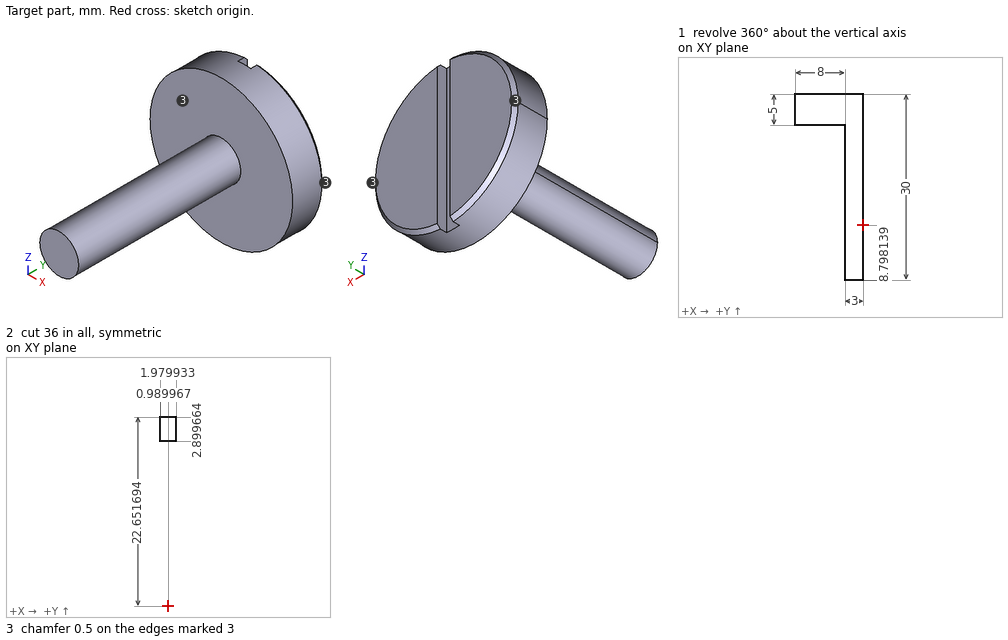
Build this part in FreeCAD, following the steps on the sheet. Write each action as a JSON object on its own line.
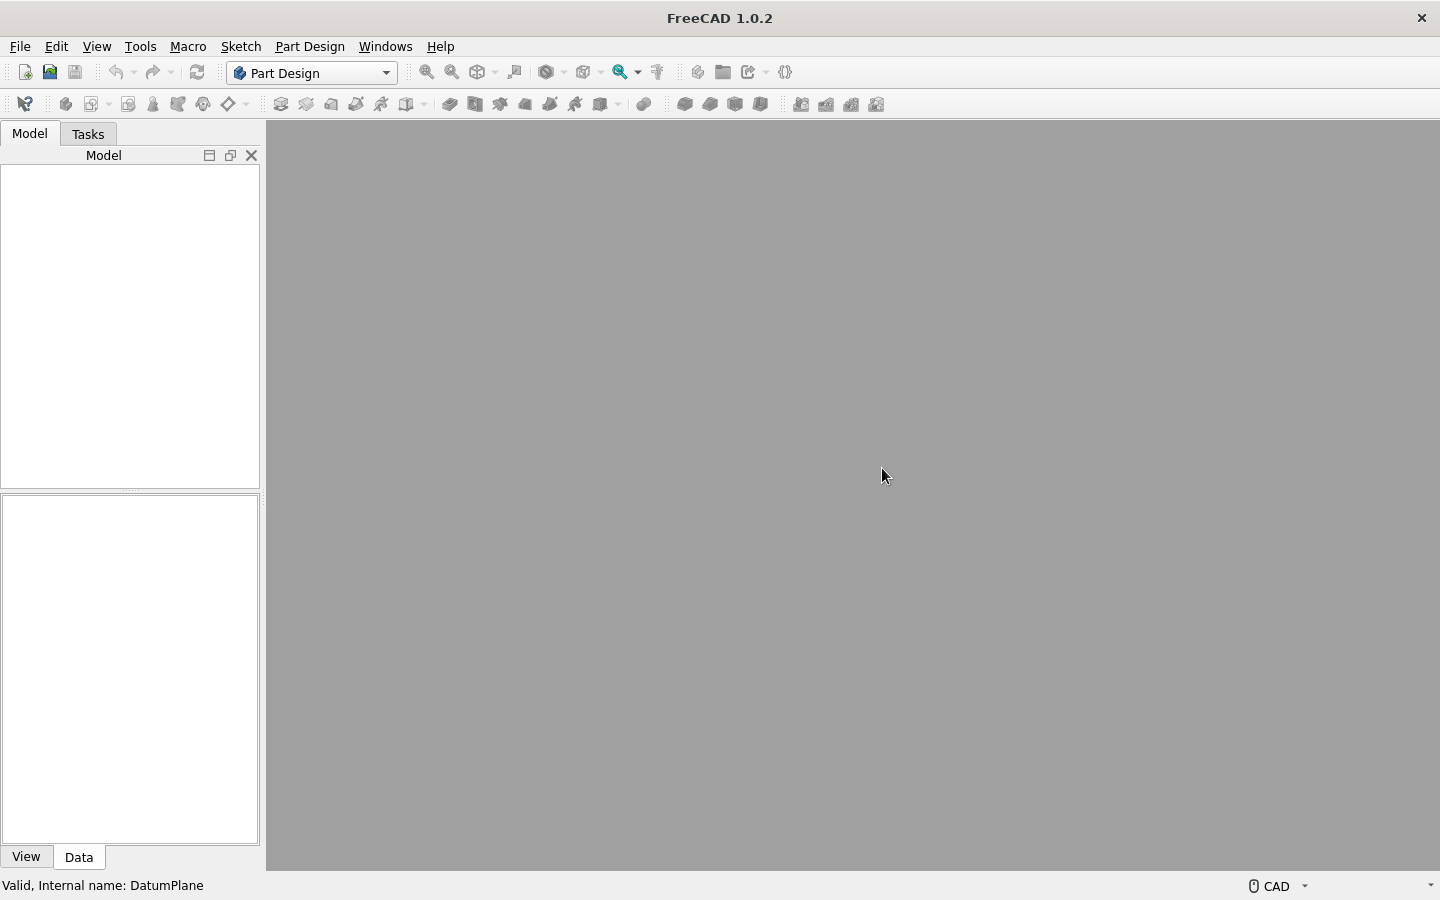
{"action": "left_click", "coordinate": [25, 72]}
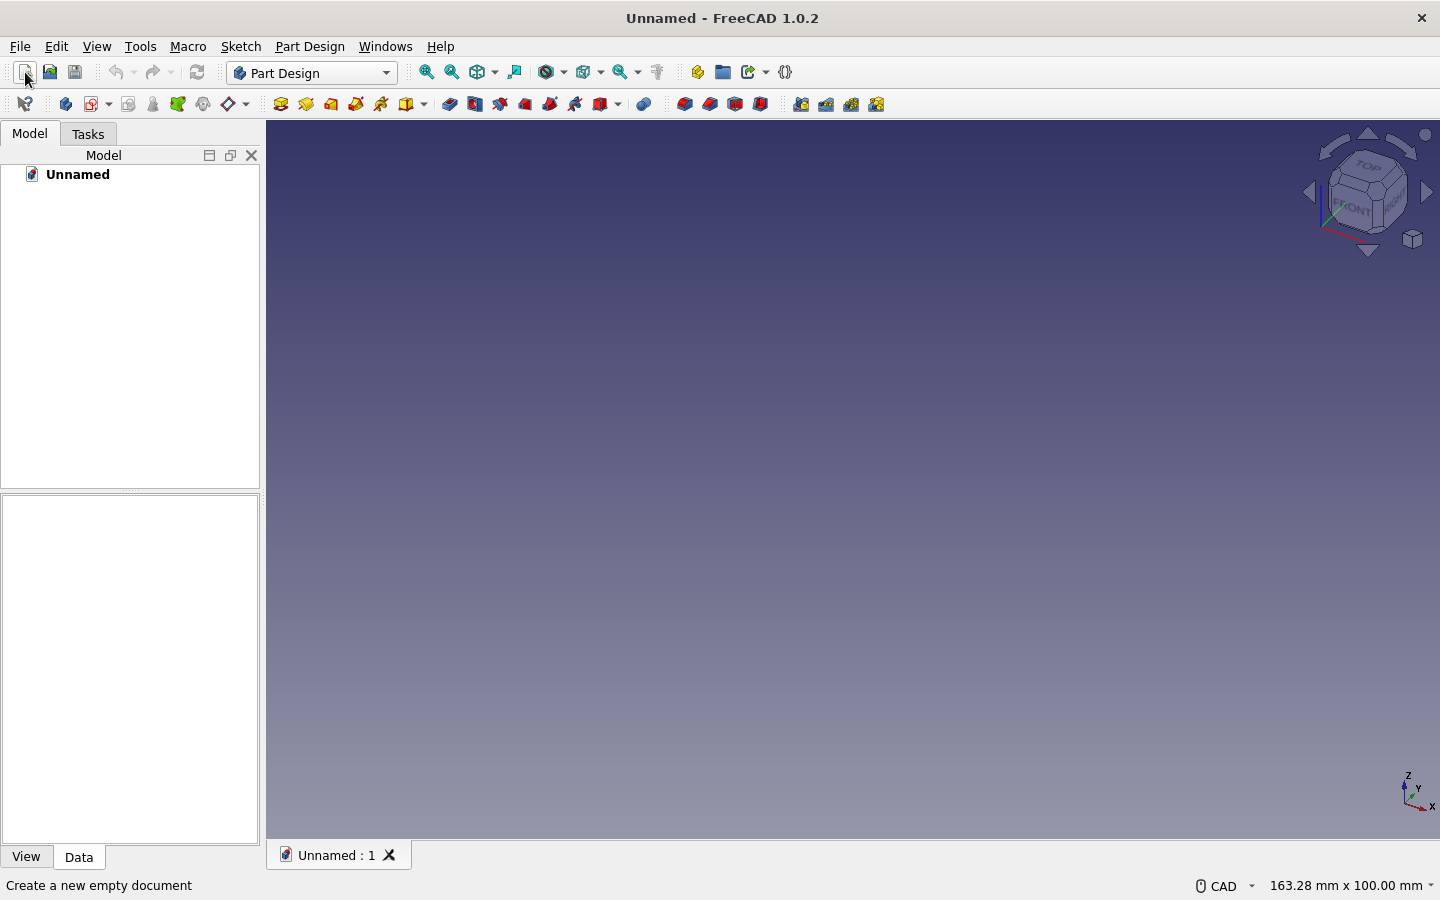
{"action": "left_click", "coordinate": [90, 104]}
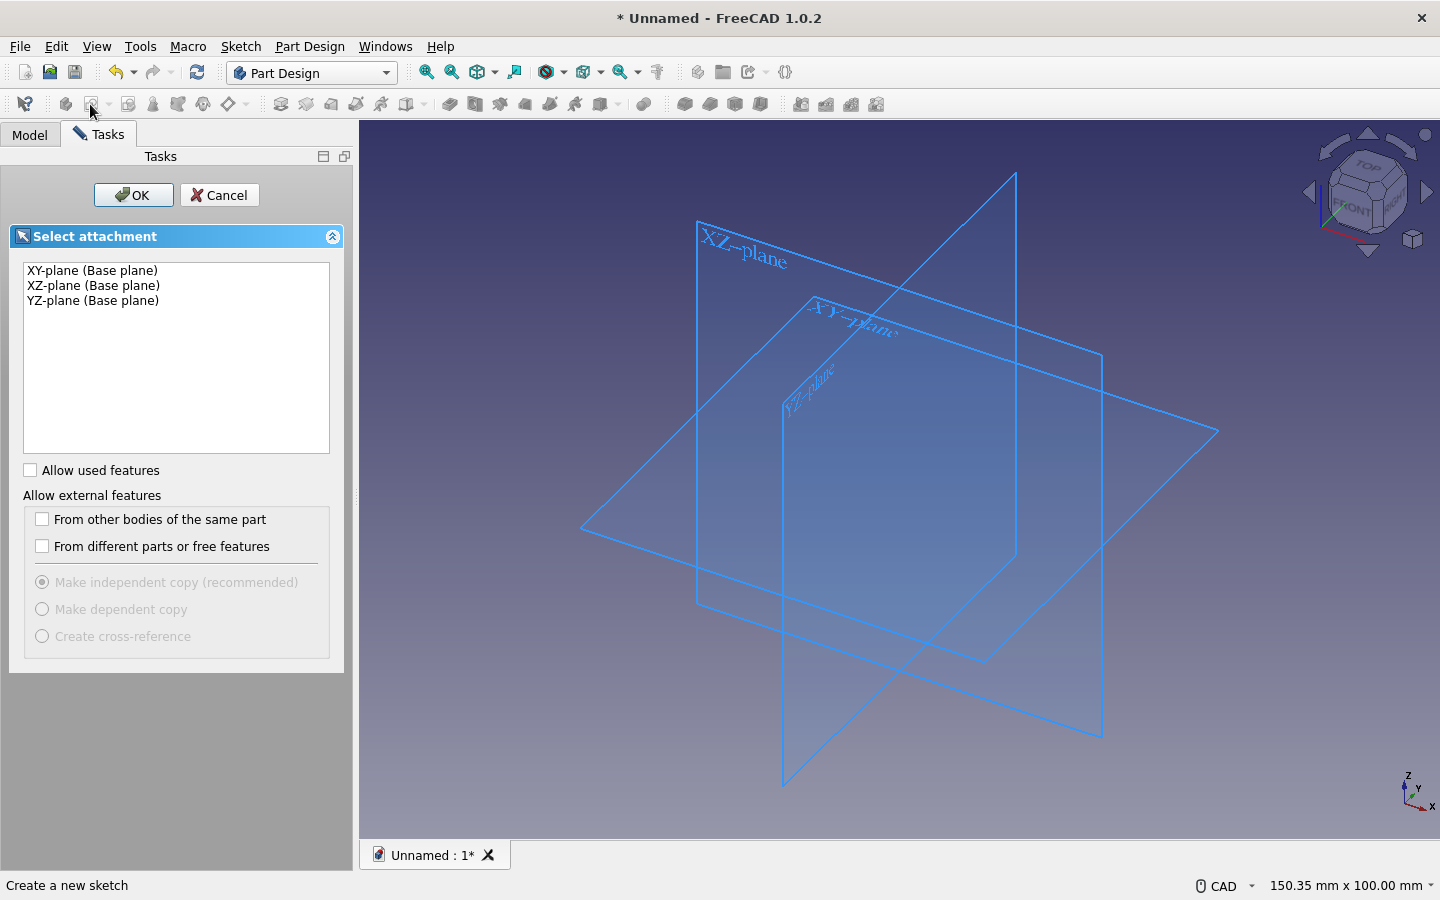
{"action": "left_click", "coordinate": [84, 270]}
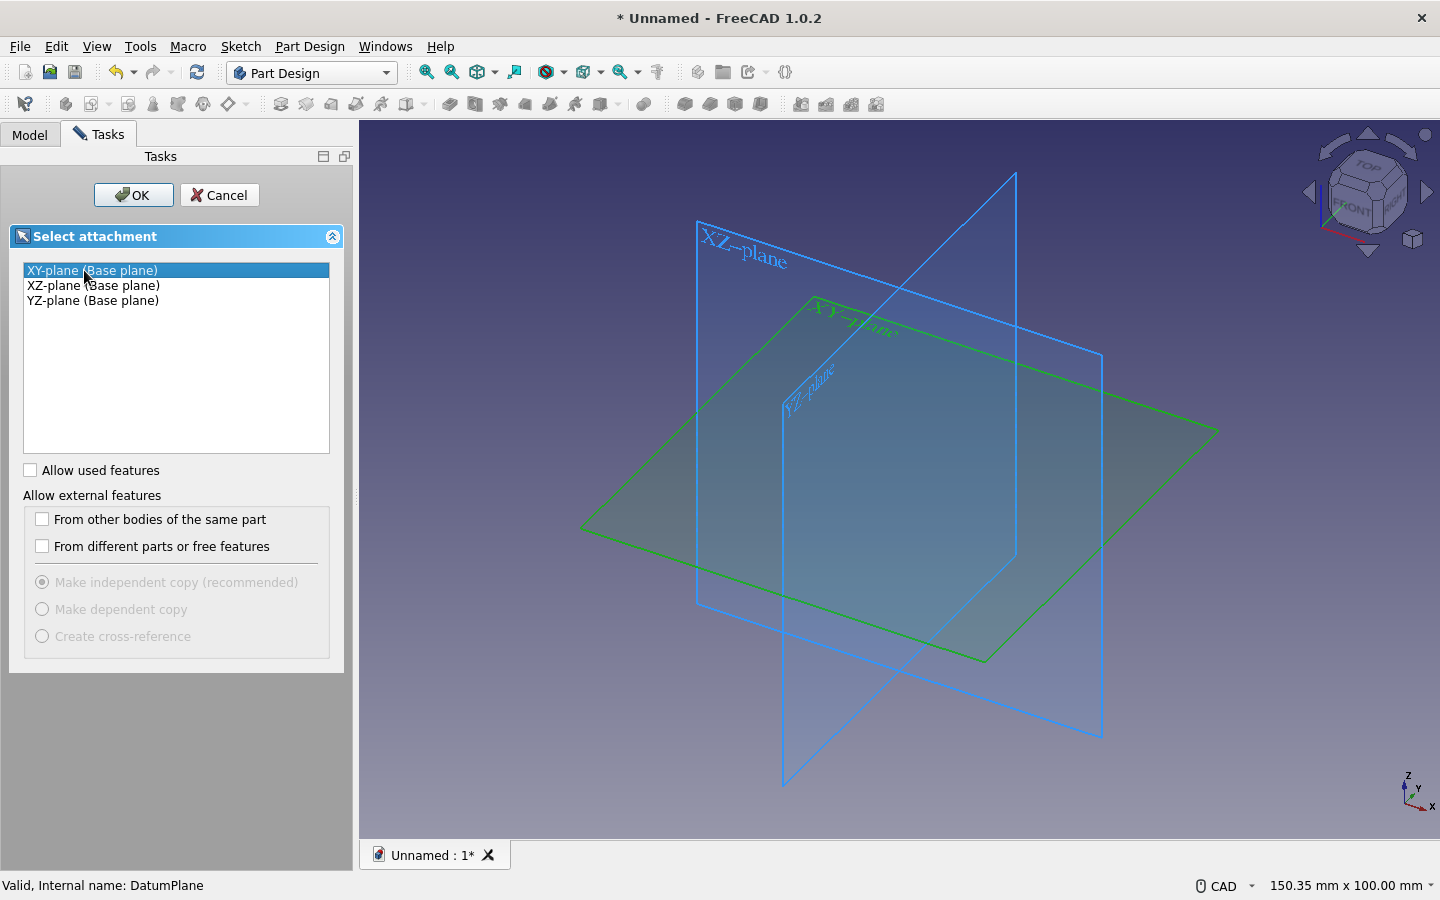
{"action": "left_click", "coordinate": [134, 195]}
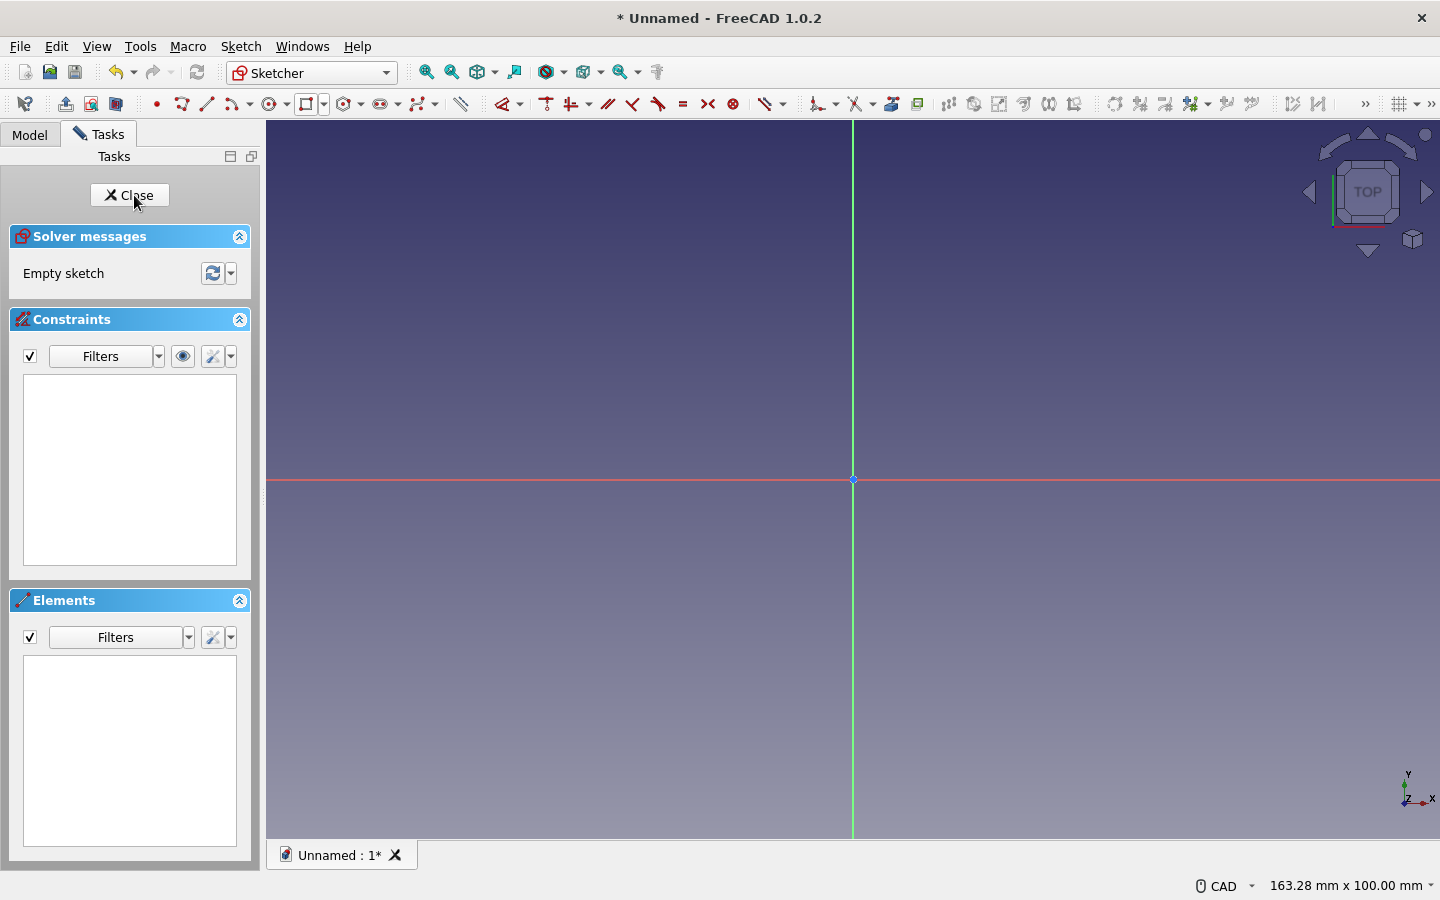
{"action": "scroll", "coordinate": [837, 399], "scroll_direction": "up", "scroll_amount": 4}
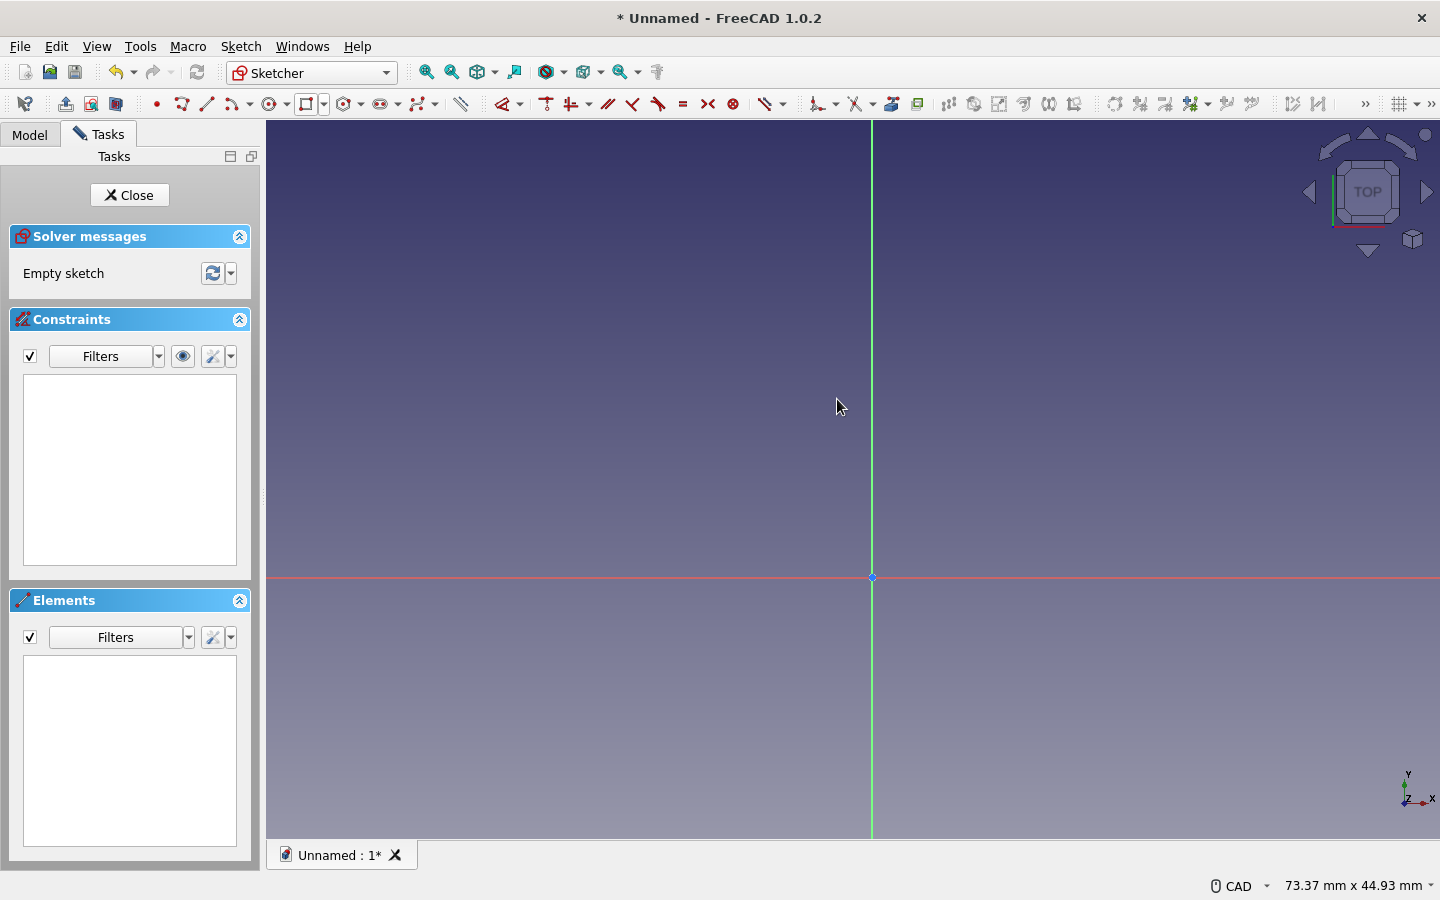
{"action": "left_click", "coordinate": [182, 104]}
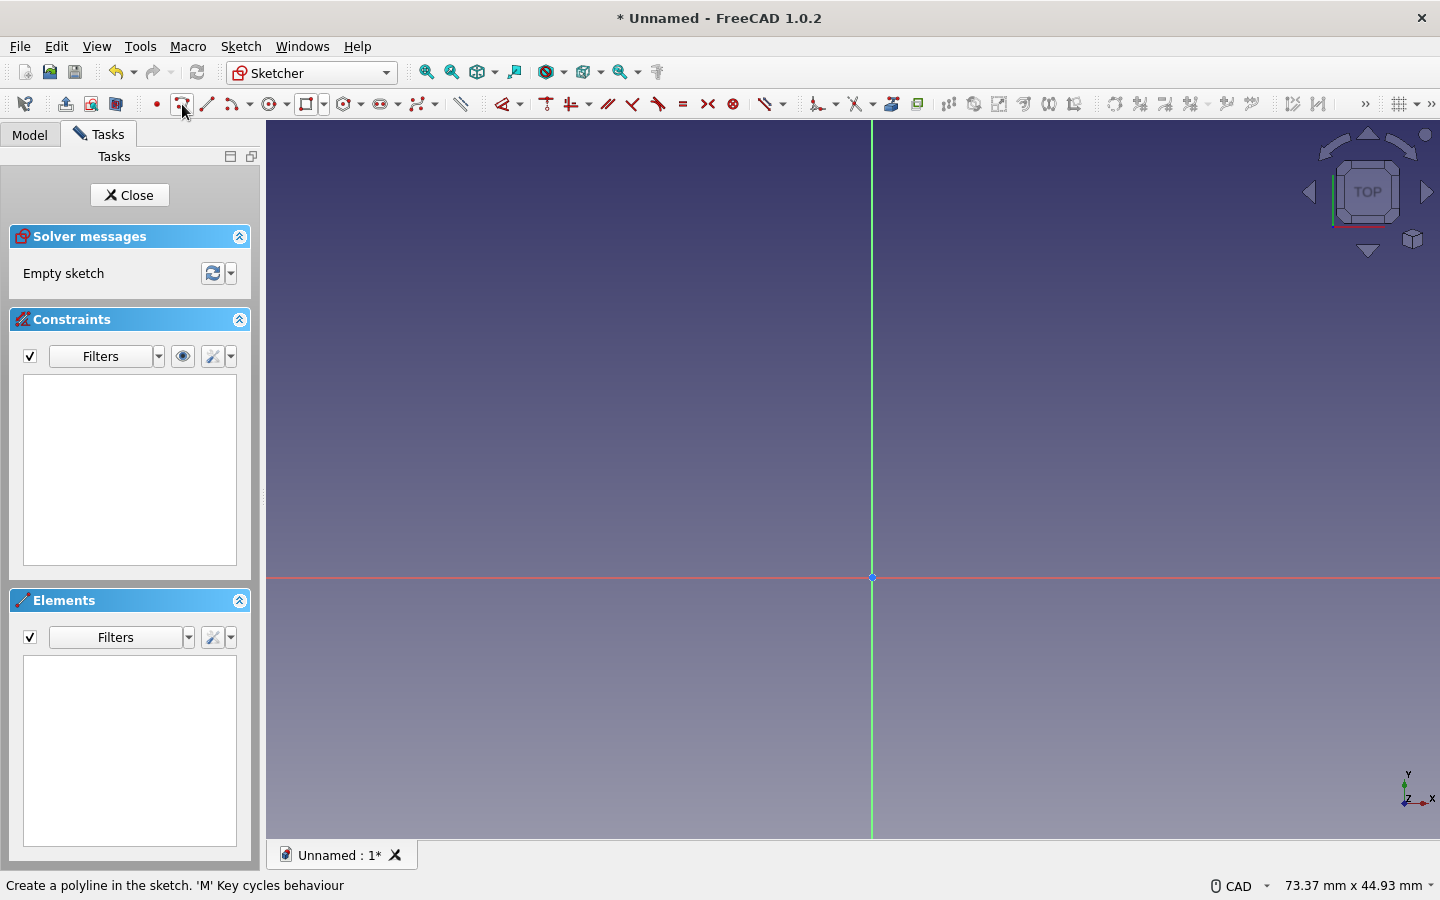
{"action": "left_click", "coordinate": [872, 718]}
{"action": "left_click", "coordinate": [863, 238]}
{"action": "left_click", "coordinate": [696, 238]}
{"action": "left_click", "coordinate": [696, 318]}
{"action": "left_click", "coordinate": [824, 318]}
{"action": "left_click", "coordinate": [824, 718]}
{"action": "left_click", "coordinate": [872, 719]}
{"action": "key", "text": "Escape"}
{"action": "key", "text": "Escape"}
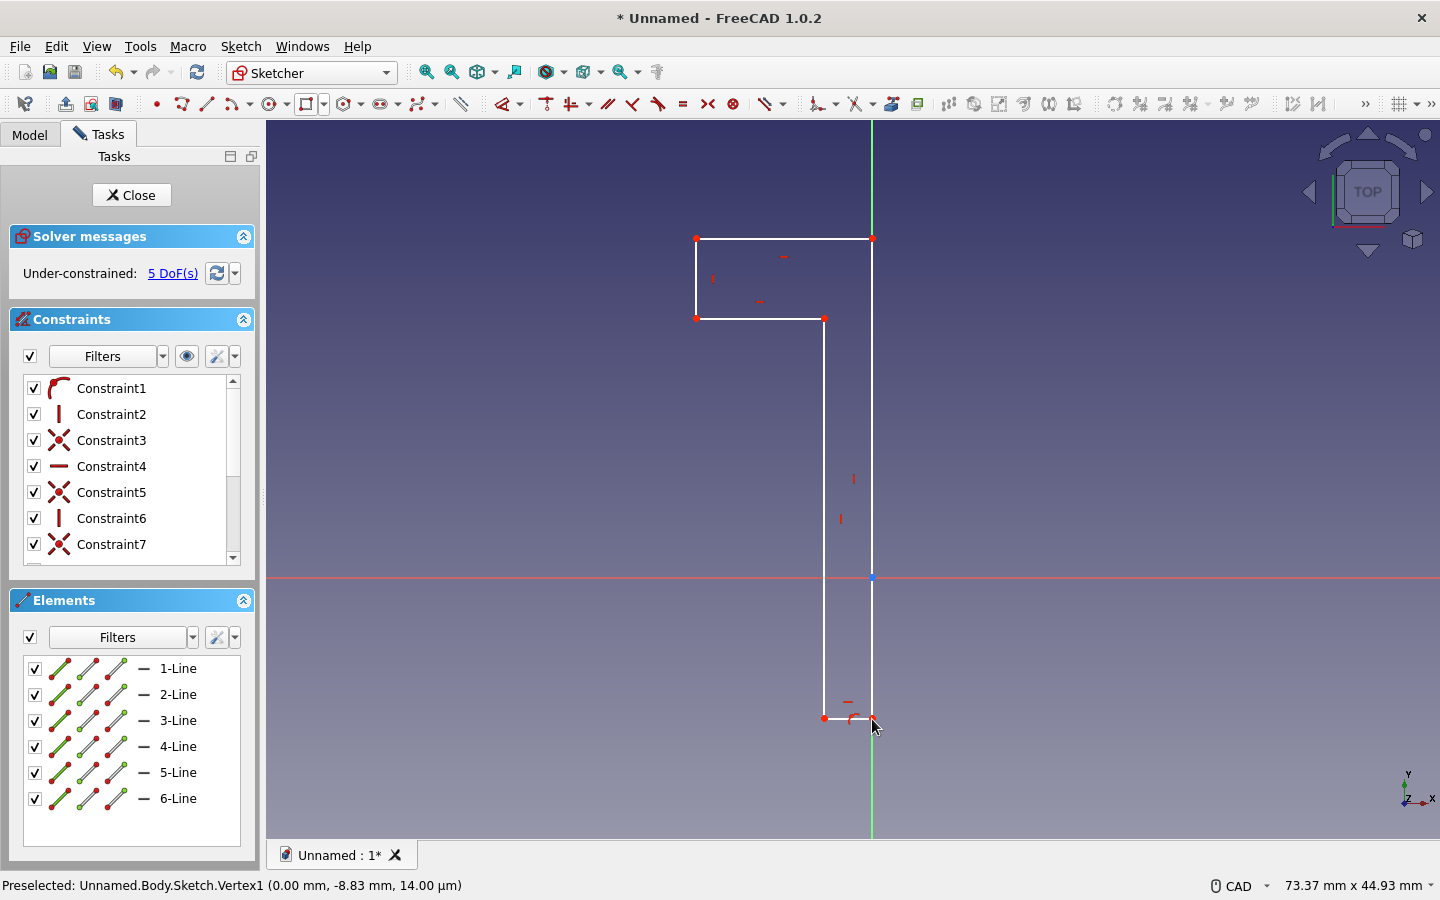
{"action": "left_click", "coordinate": [696, 263]}